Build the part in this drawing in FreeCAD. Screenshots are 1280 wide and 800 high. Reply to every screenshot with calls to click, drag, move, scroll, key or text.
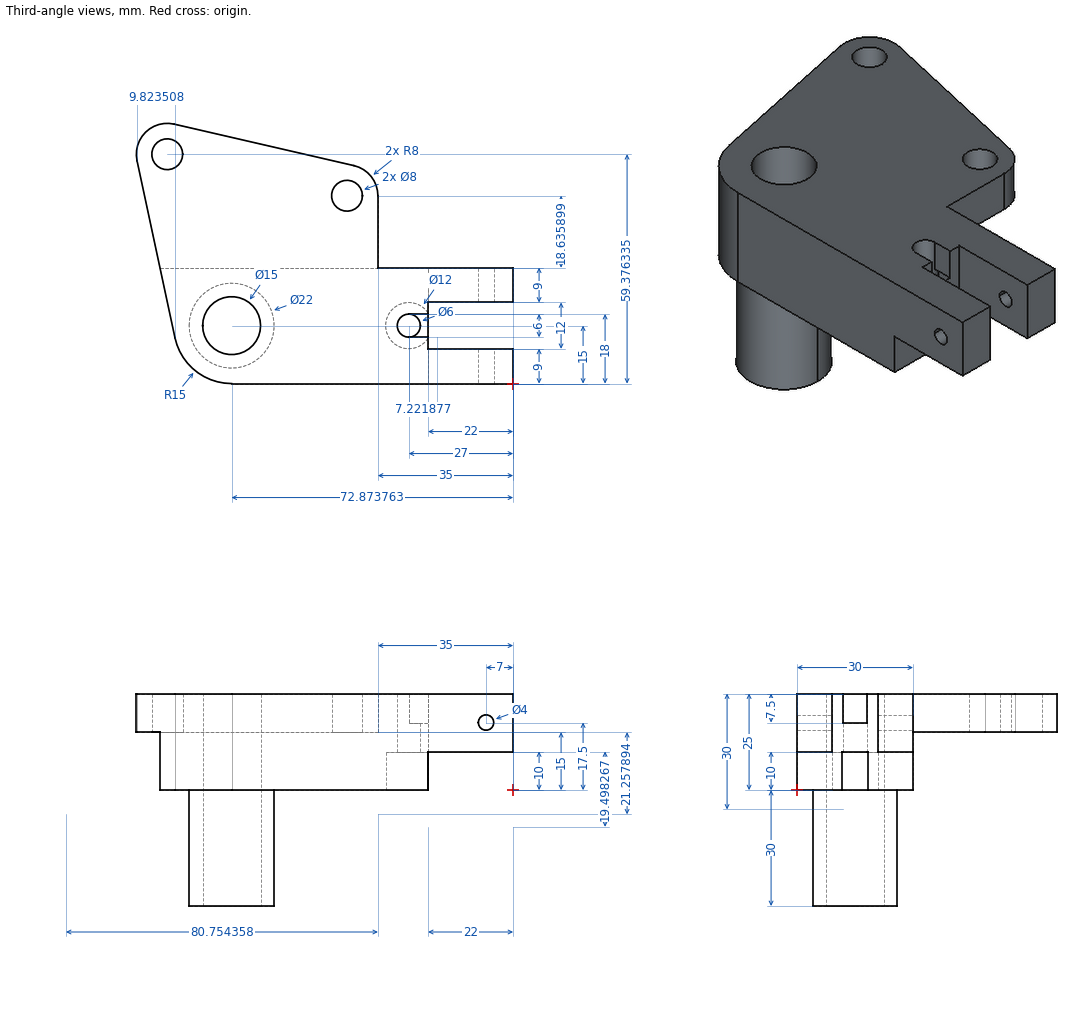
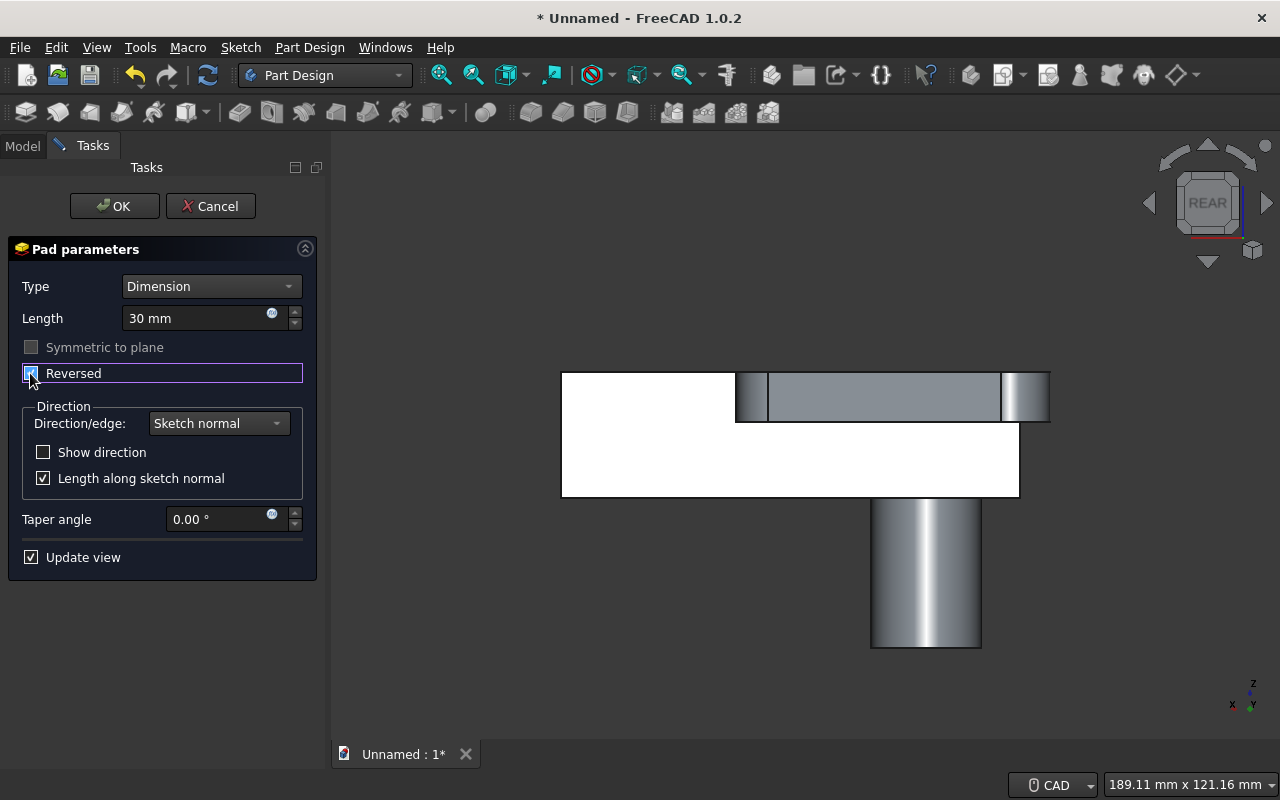
click(115, 206)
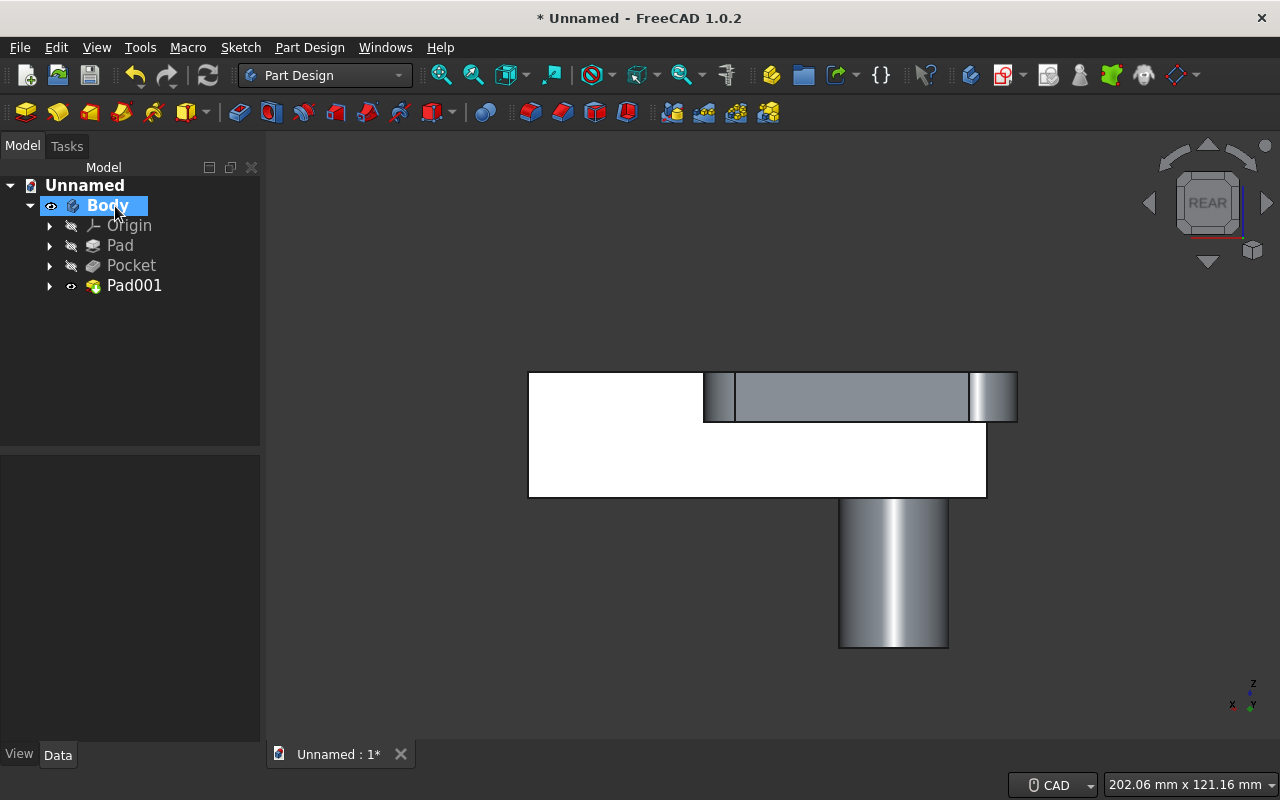
key(5)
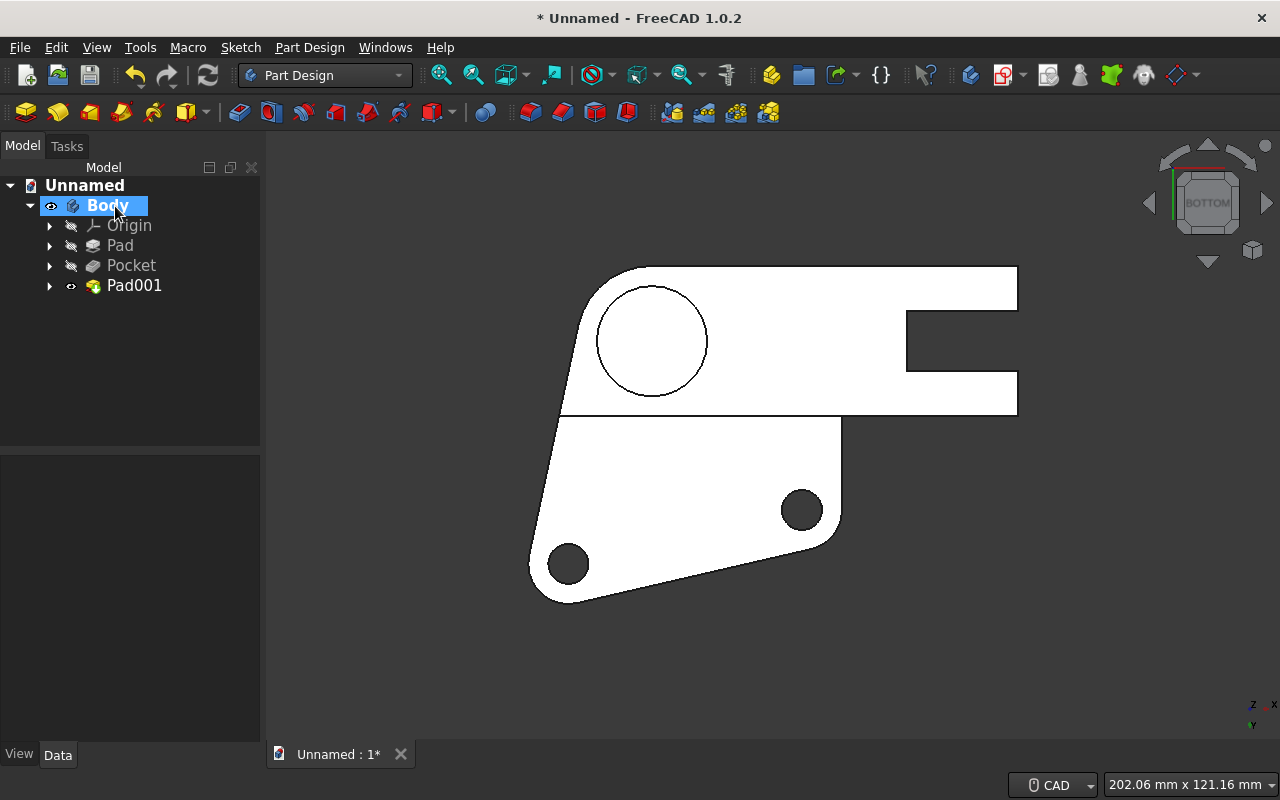
click(652, 340)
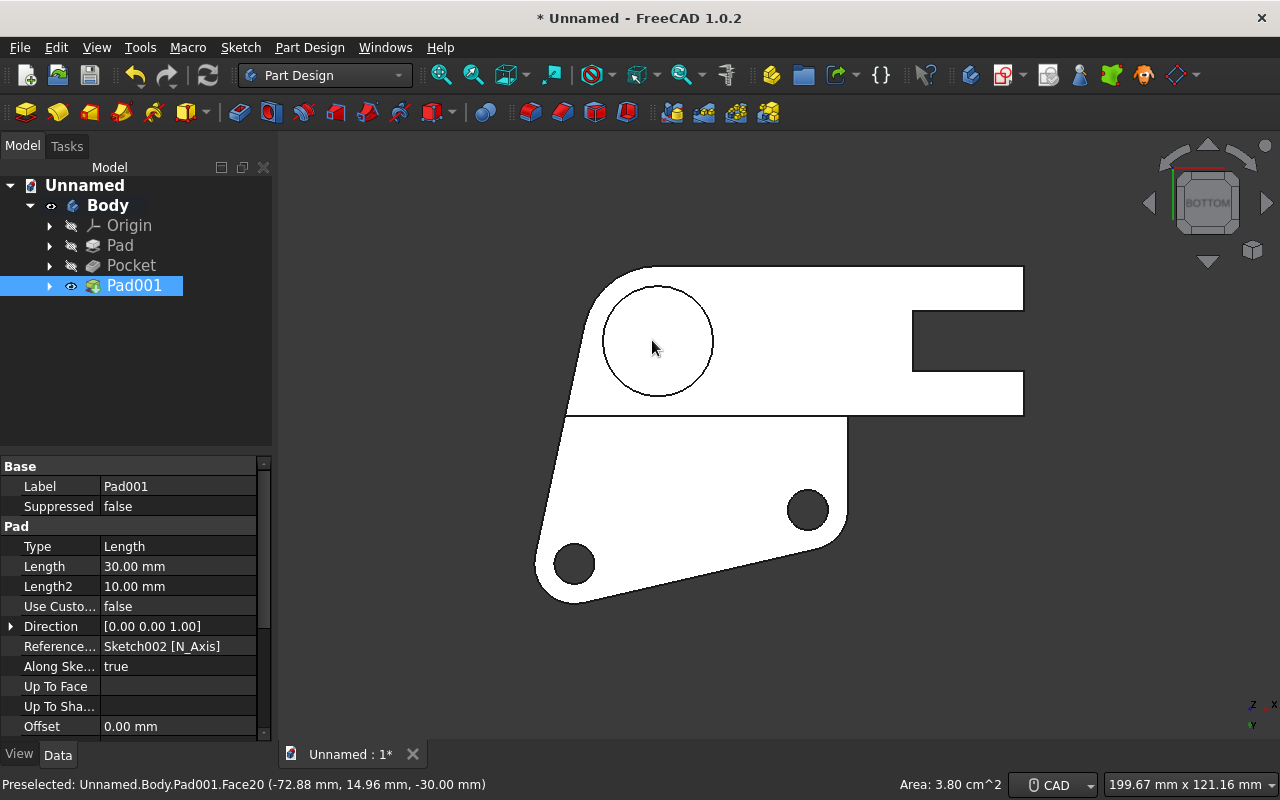
click(1004, 76)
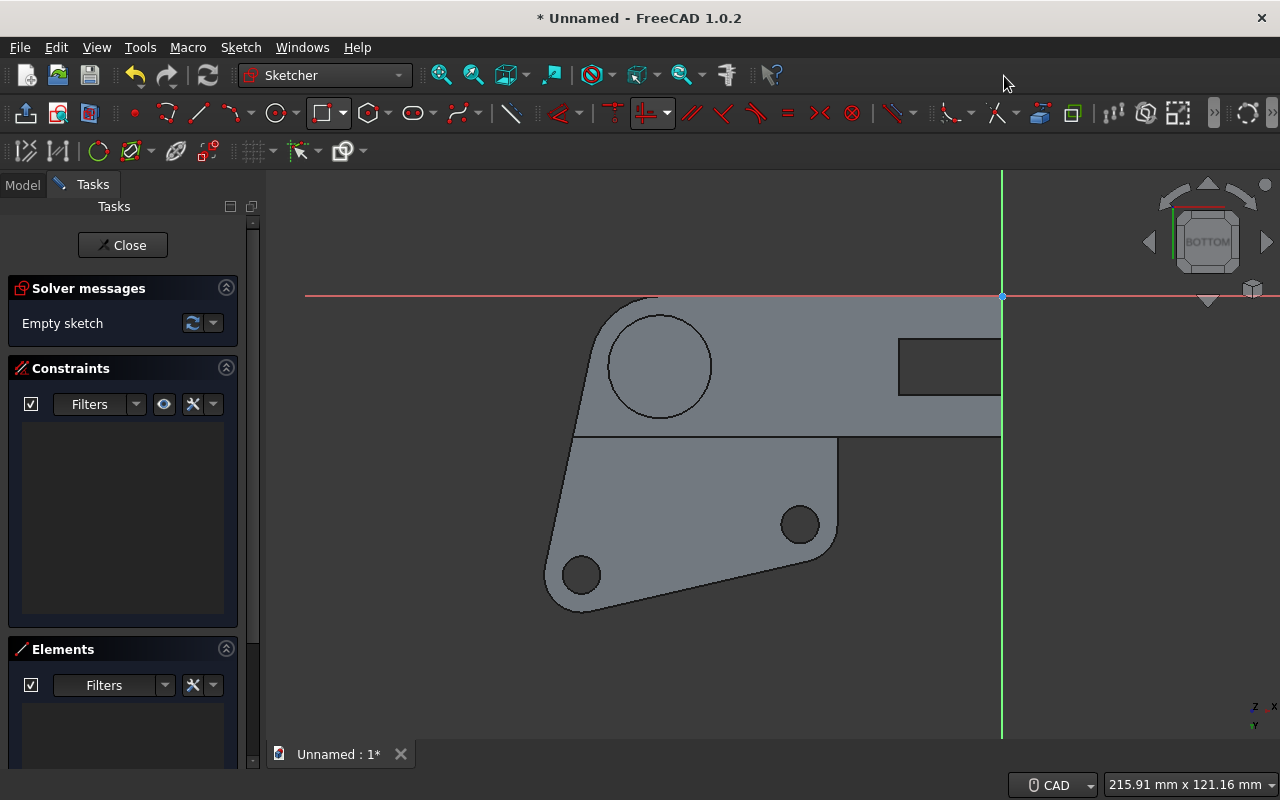
scroll(648, 345, up, 8)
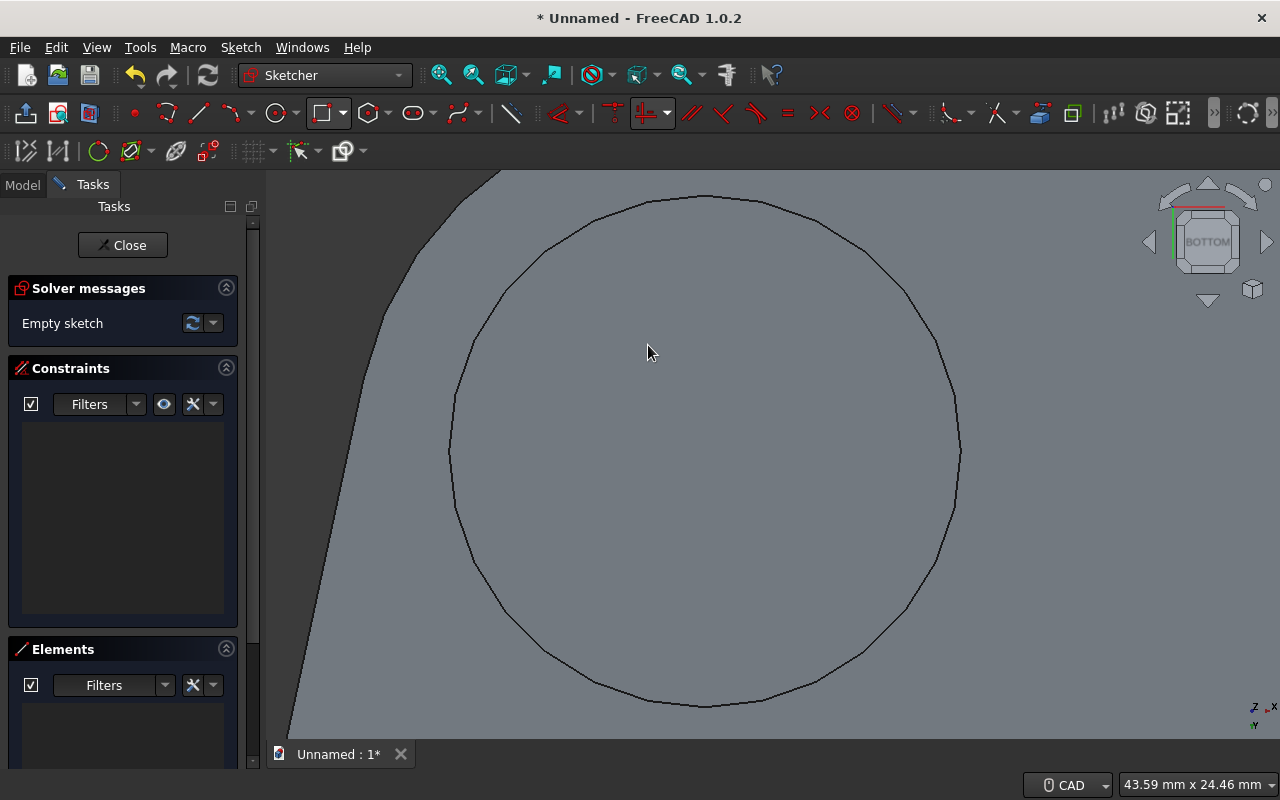
click(276, 114)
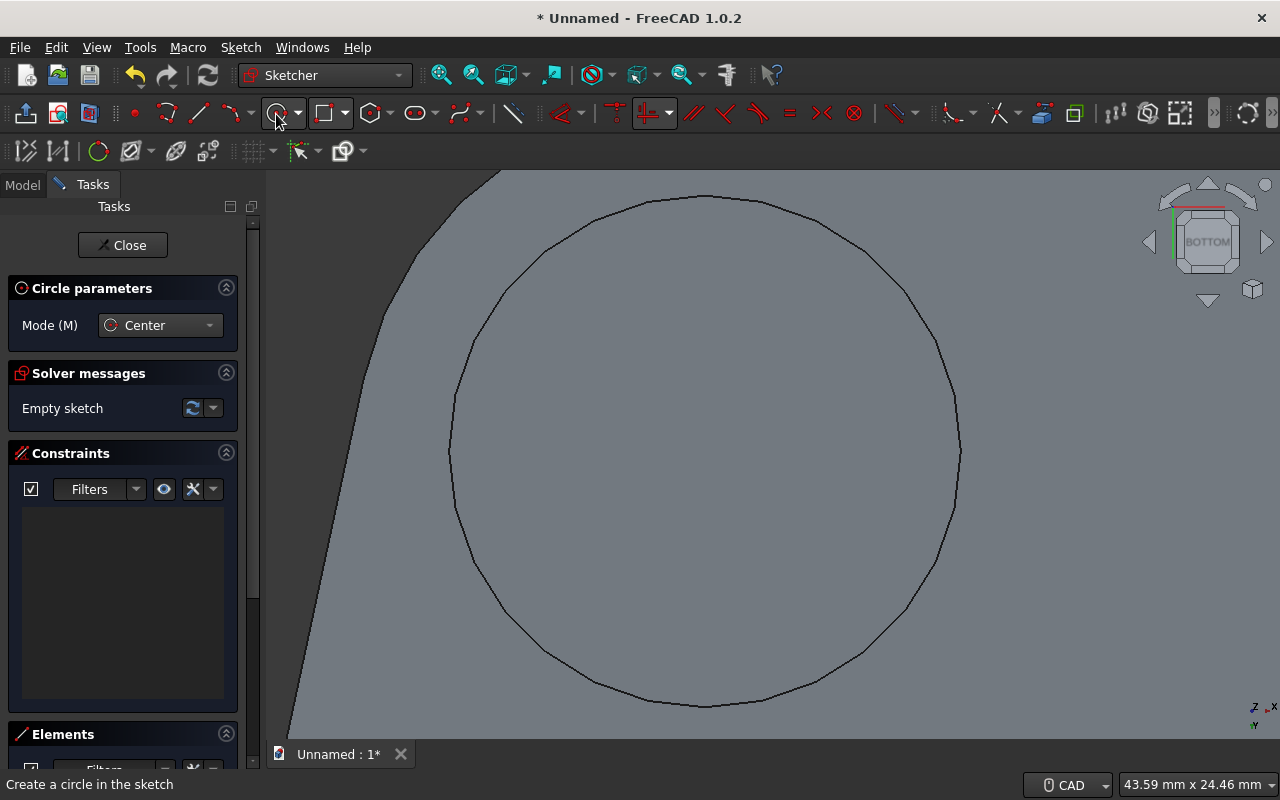
click(705, 451)
click(828, 328)
key(Escape)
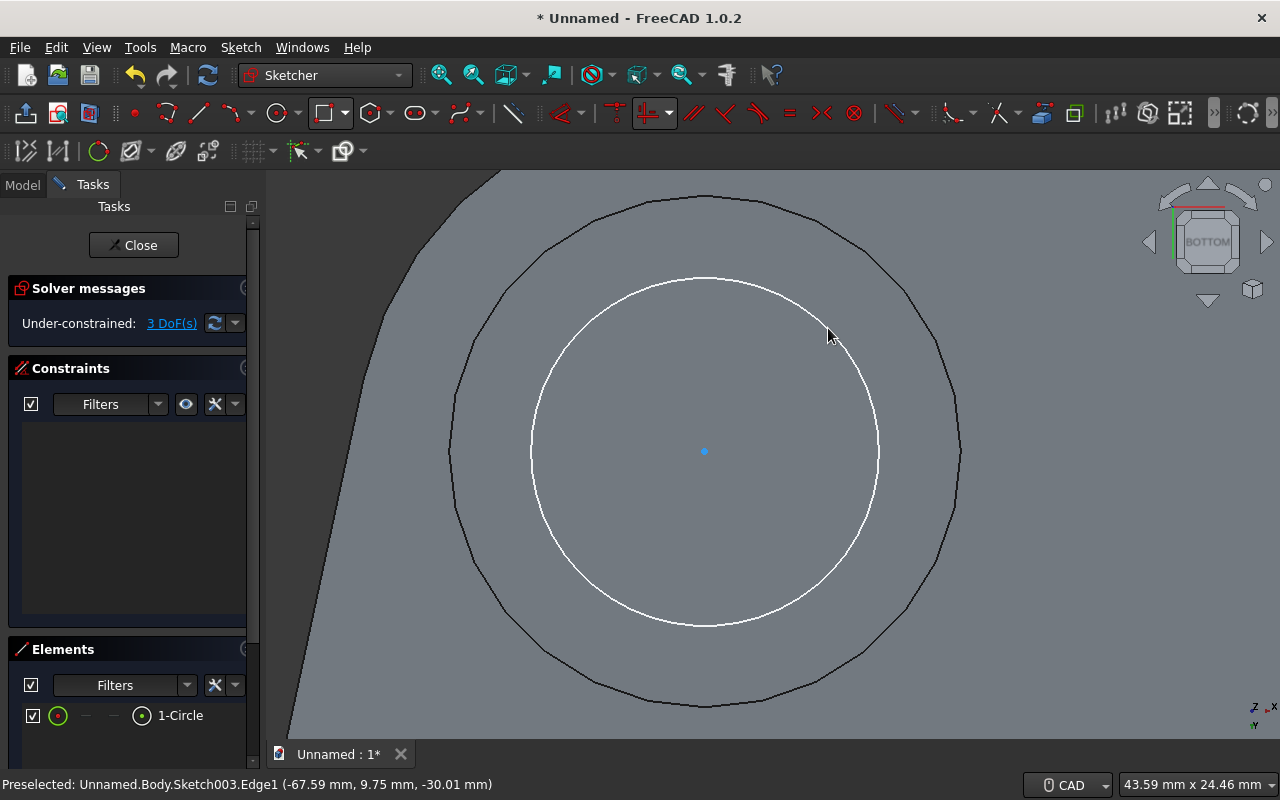
click(560, 114)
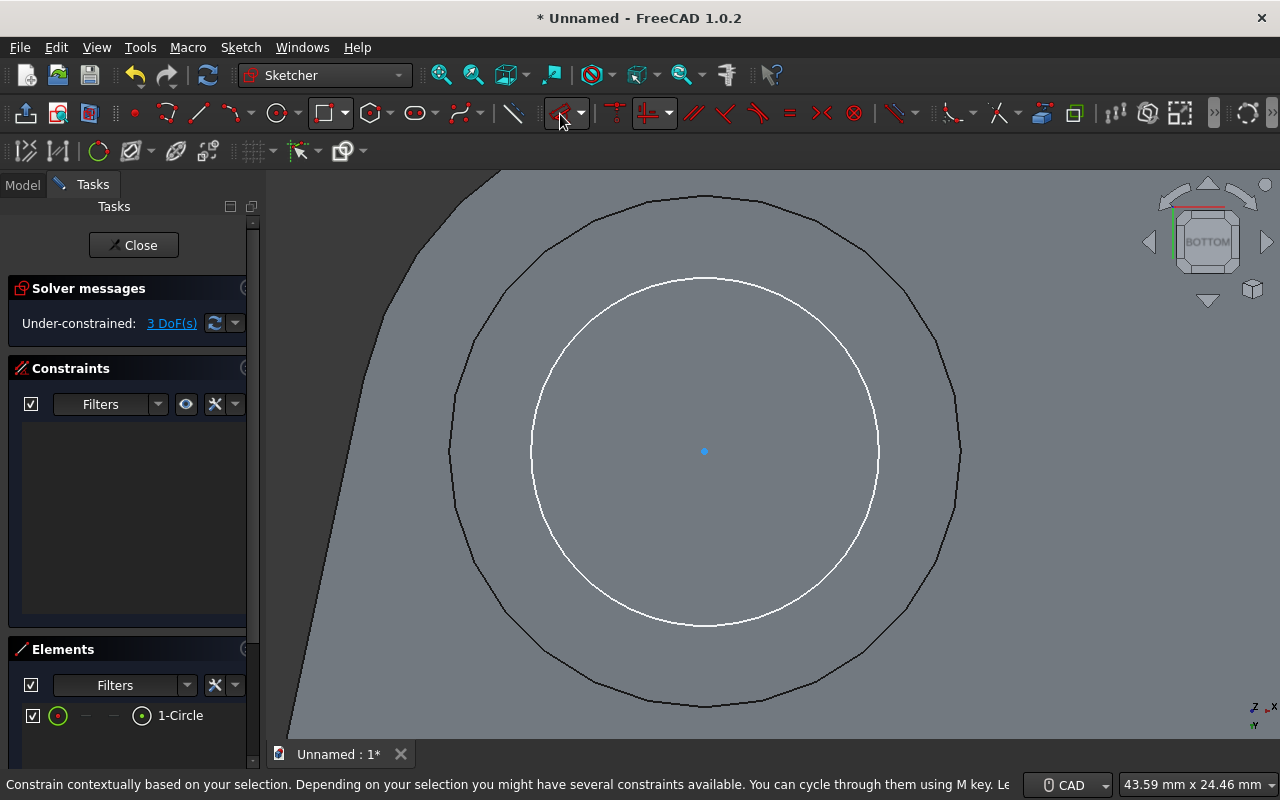
click(828, 329)
click(851, 306)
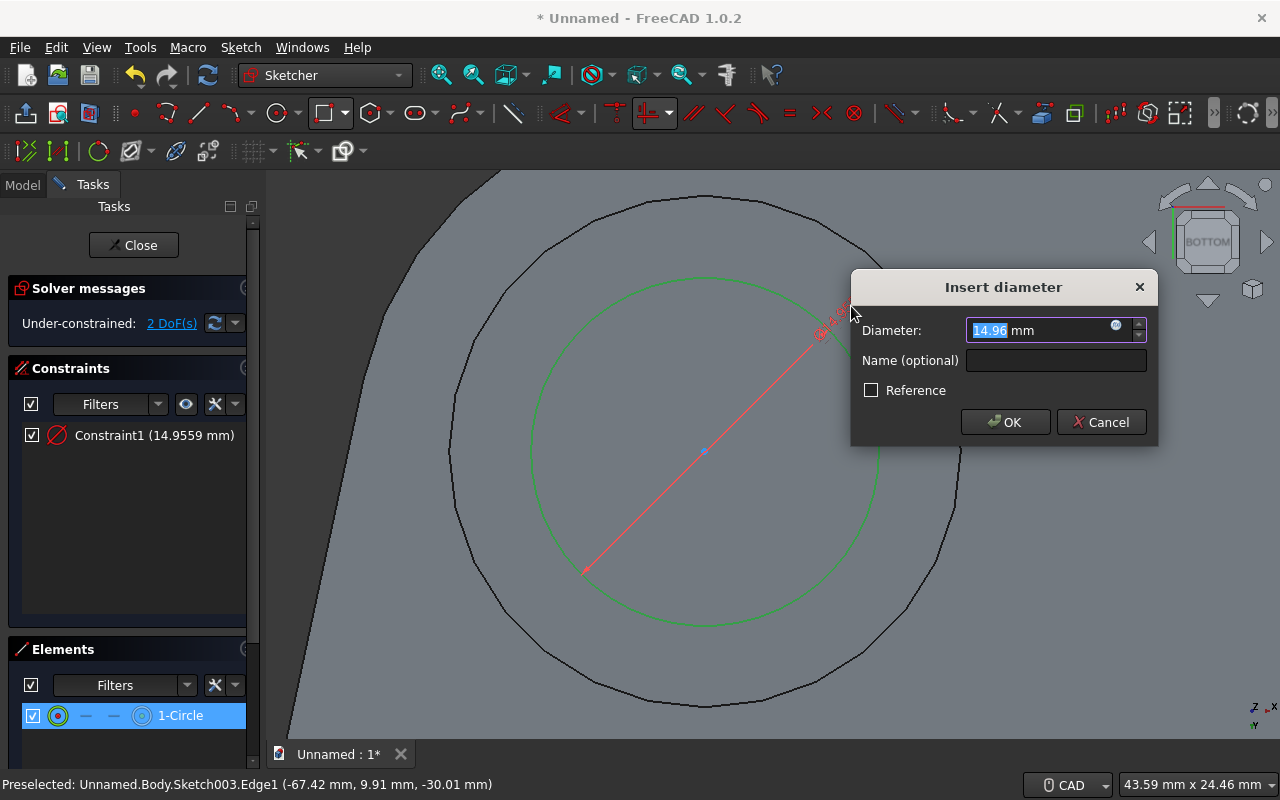
text(15)
key(Return)